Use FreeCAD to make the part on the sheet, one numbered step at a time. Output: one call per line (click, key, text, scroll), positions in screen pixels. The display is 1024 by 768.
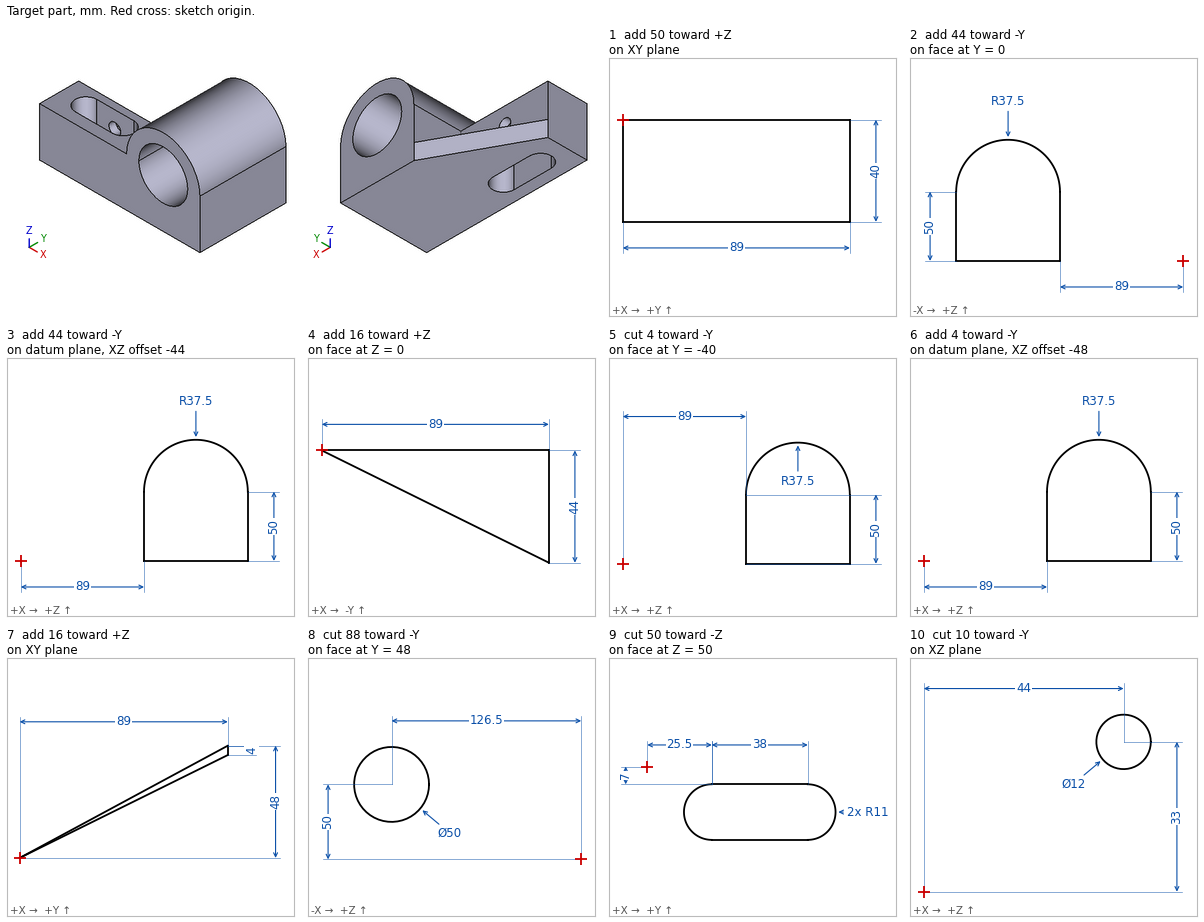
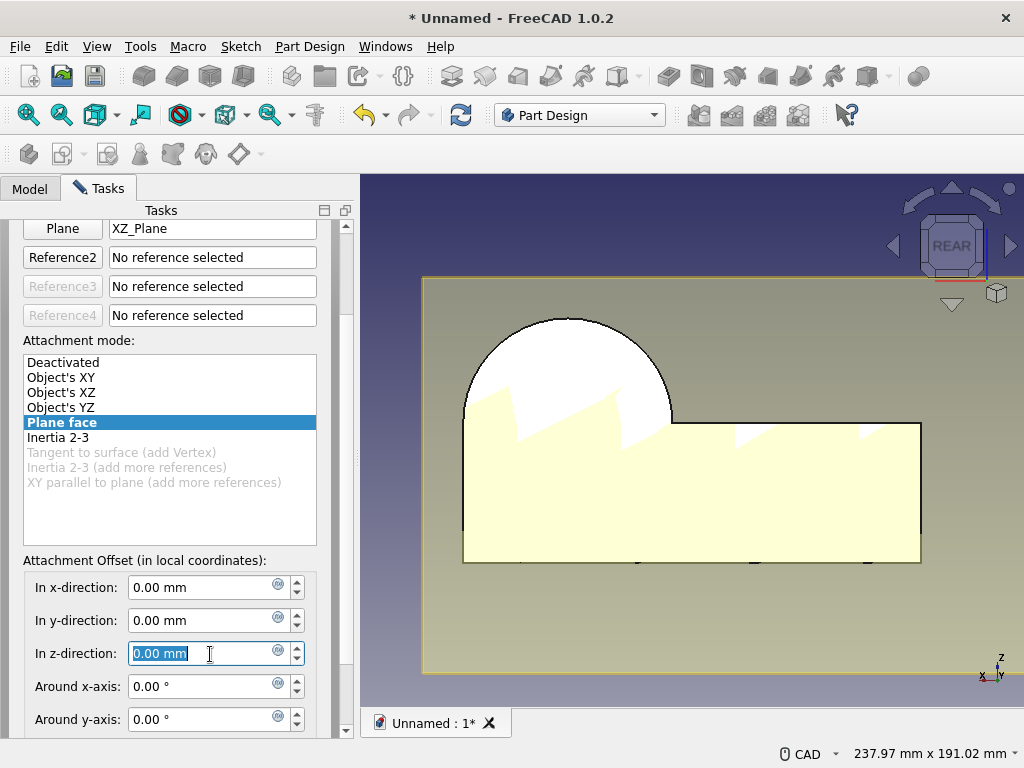
text(-44)
key(Tab)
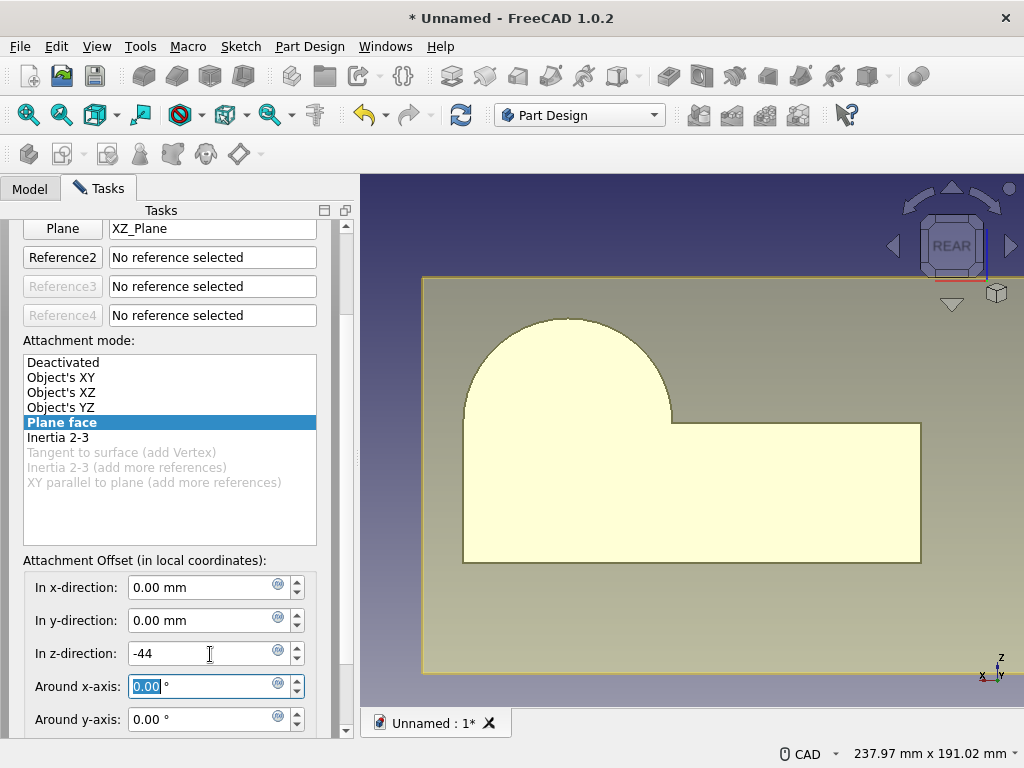
scroll(346, 479, up, 3)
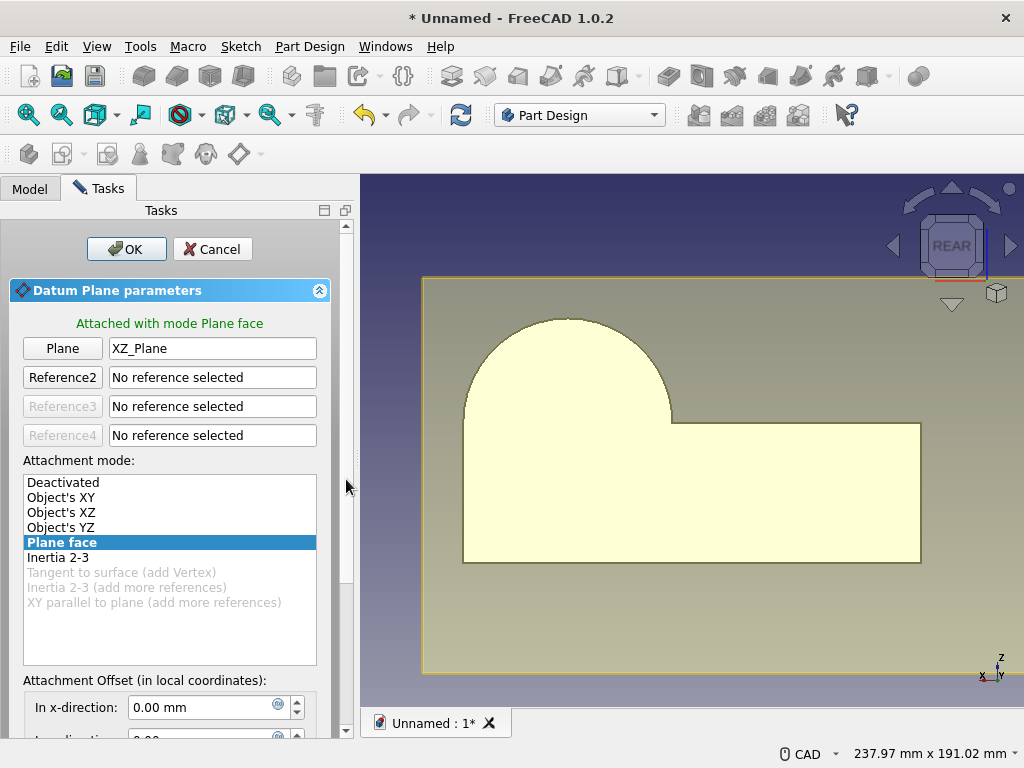
click(127, 249)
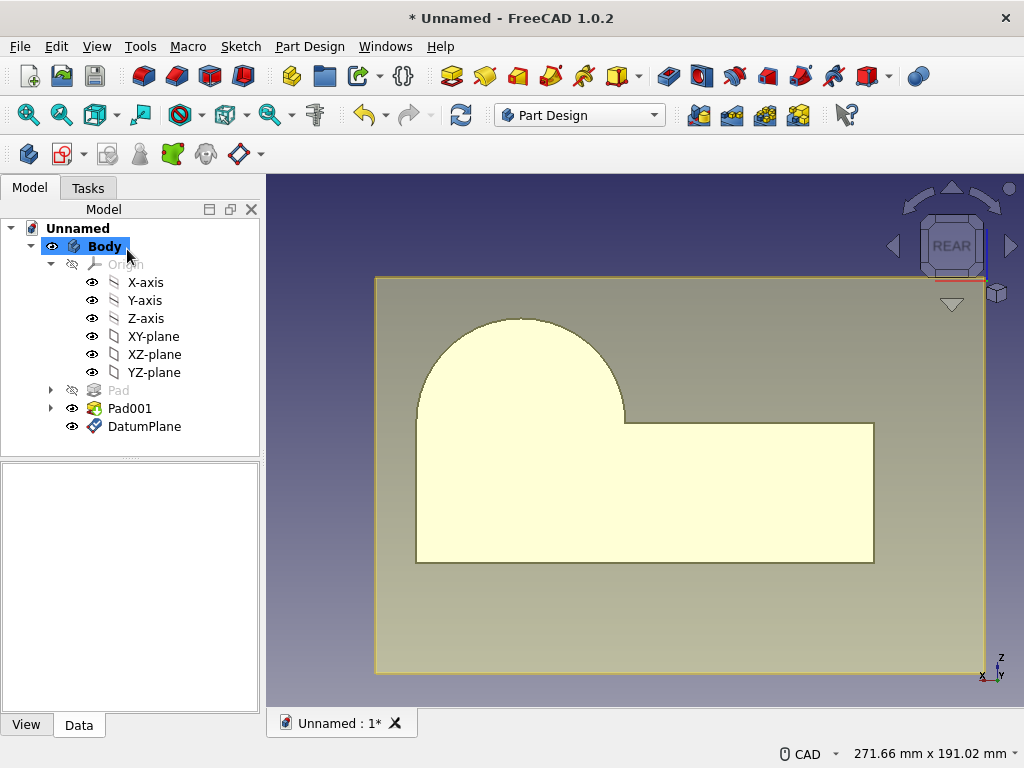
click(117, 426)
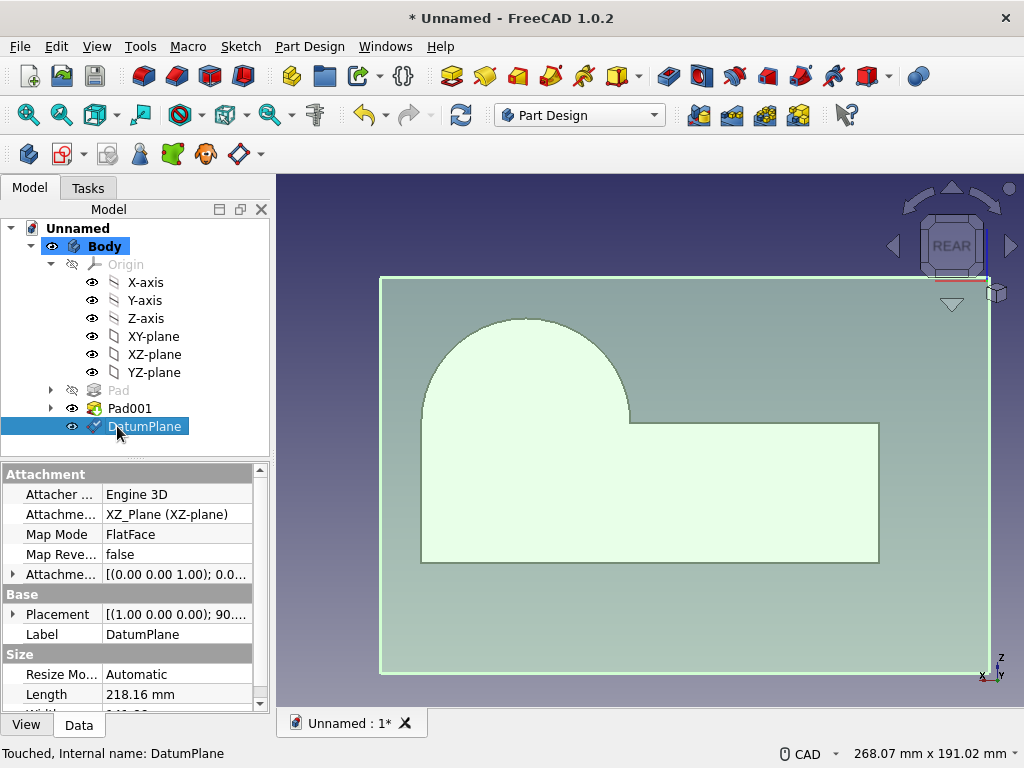
click(62, 154)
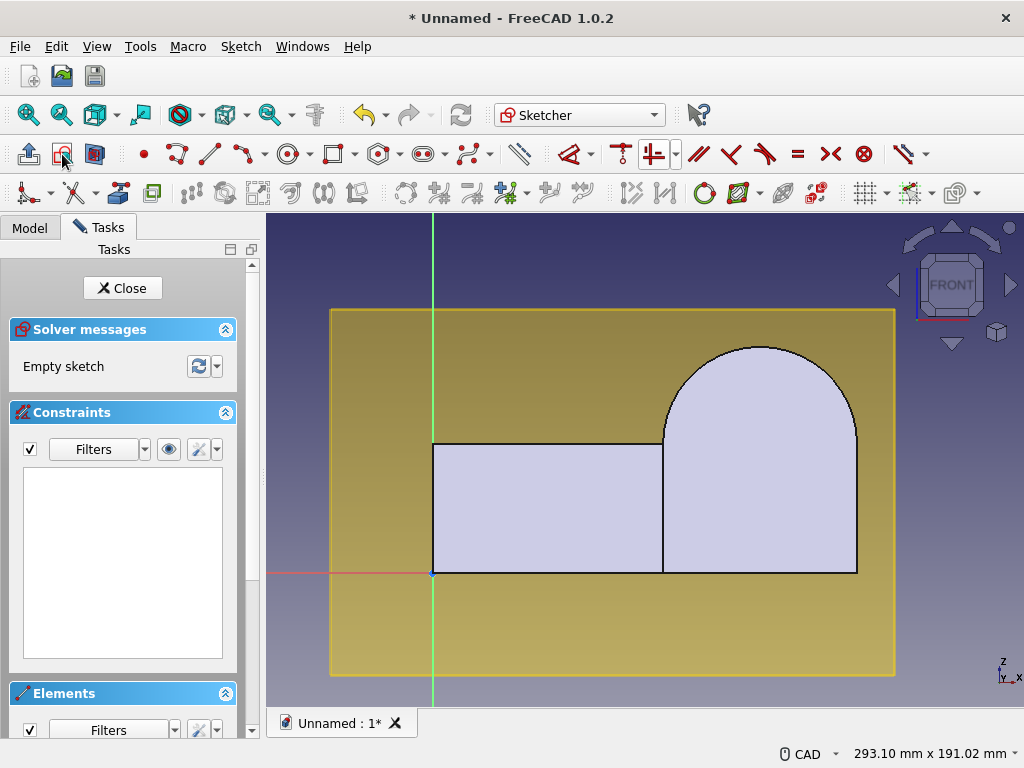
click(95, 154)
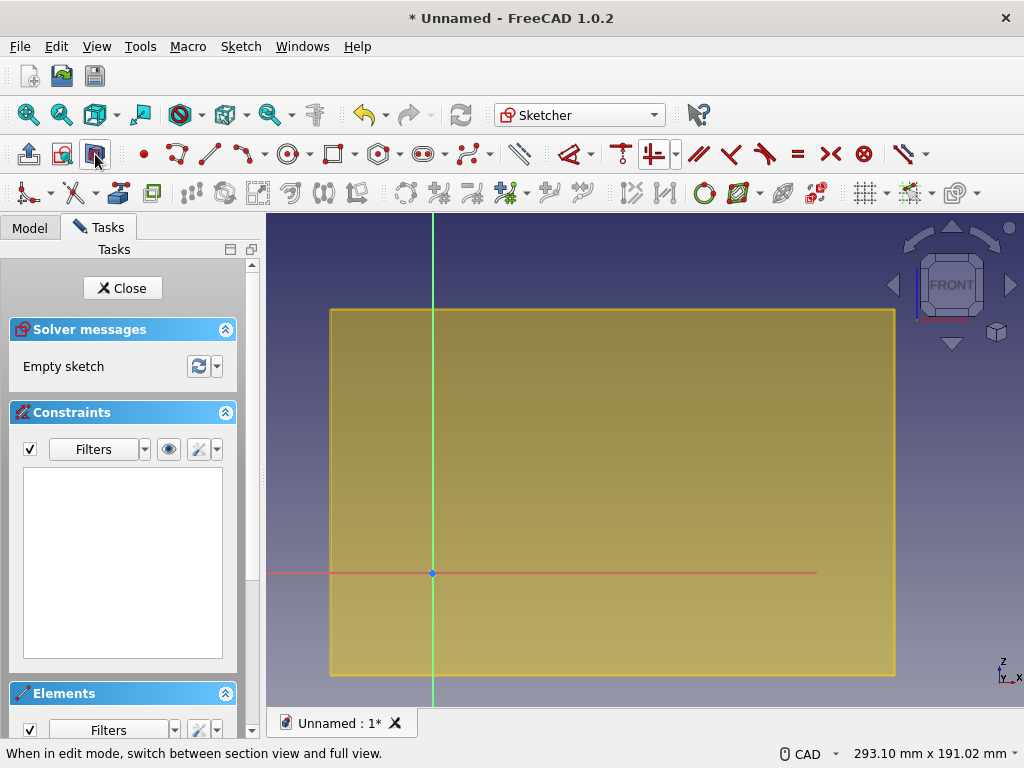
scroll(294, 460, down, 1)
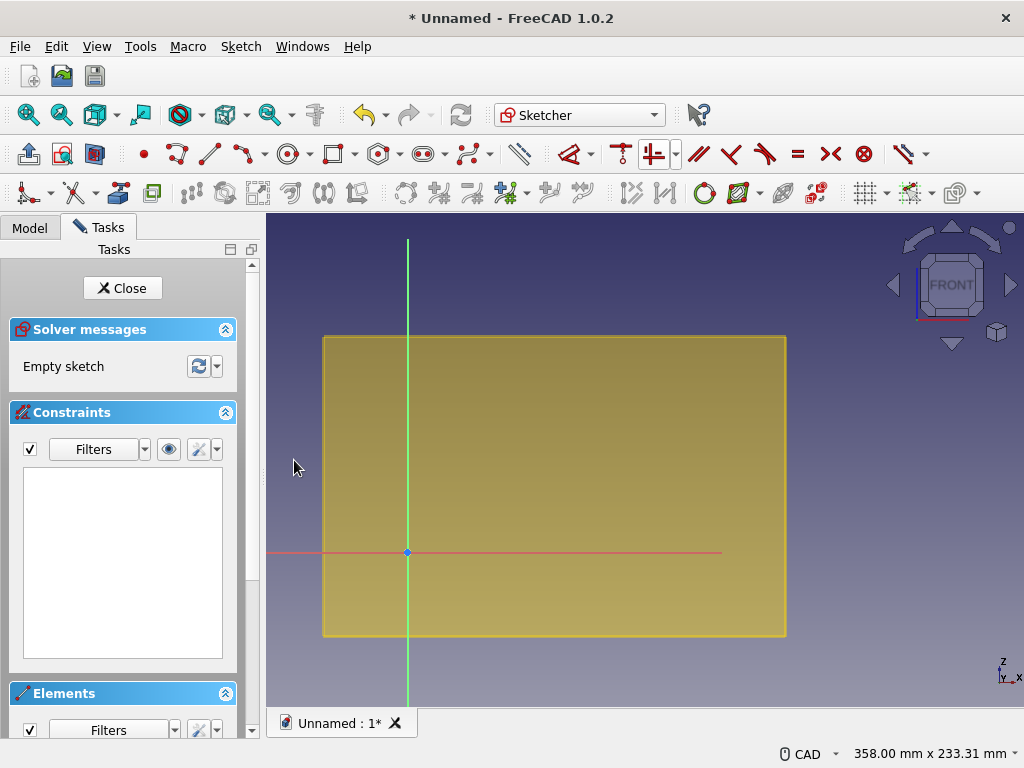
click(177, 154)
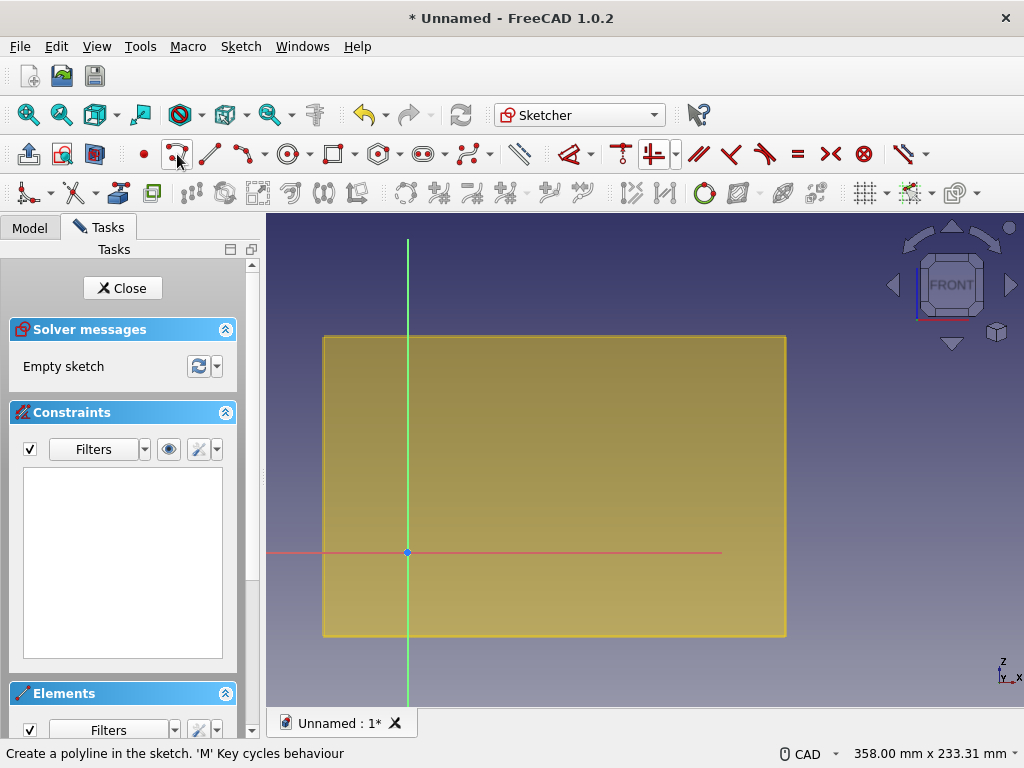
click(755, 447)
click(755, 553)
click(596, 544)
click(596, 447)
right_click(596, 447)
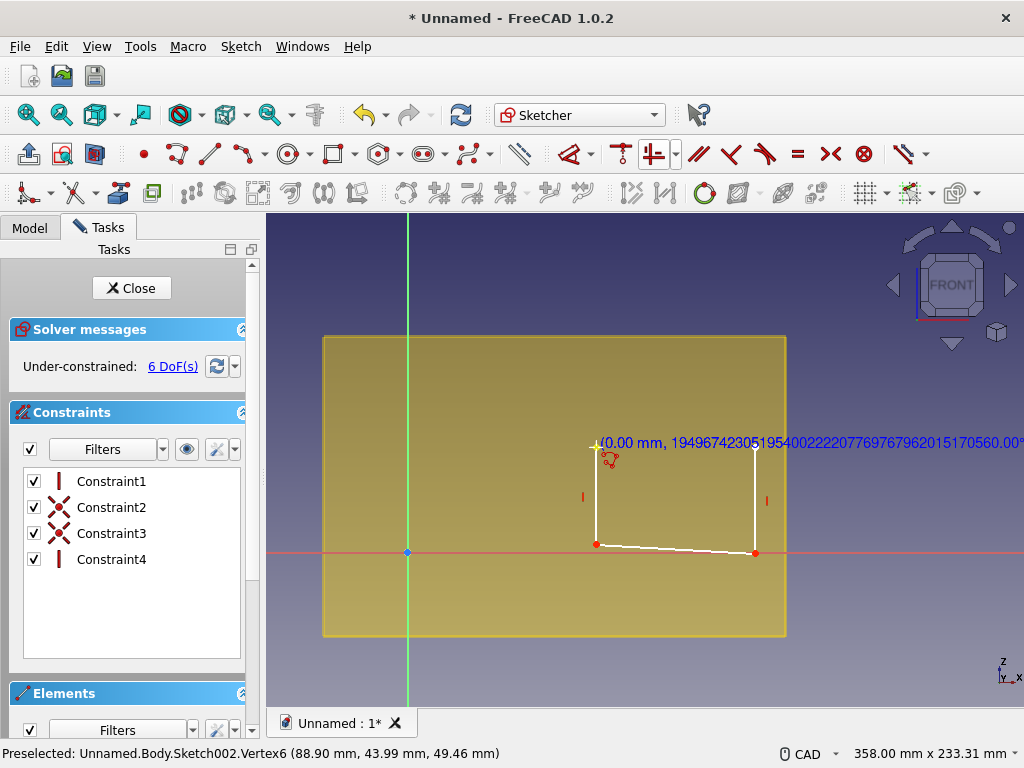
key(g)
key(3)
key(a)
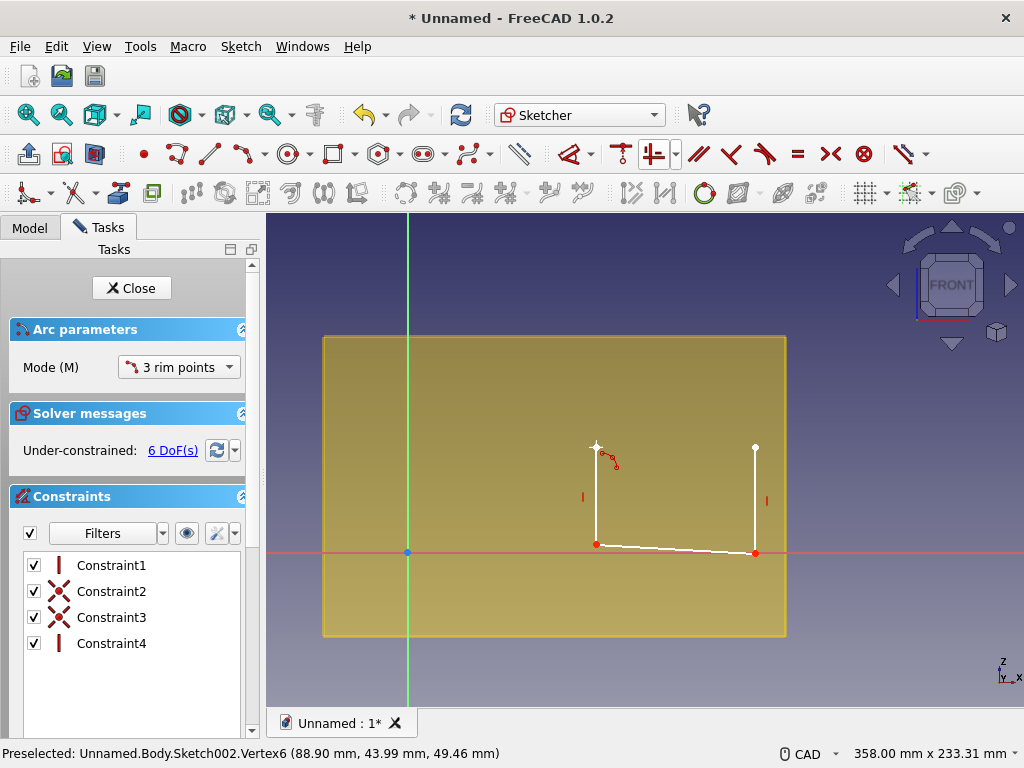
click(596, 448)
click(755, 448)
click(676, 367)
key(Escape)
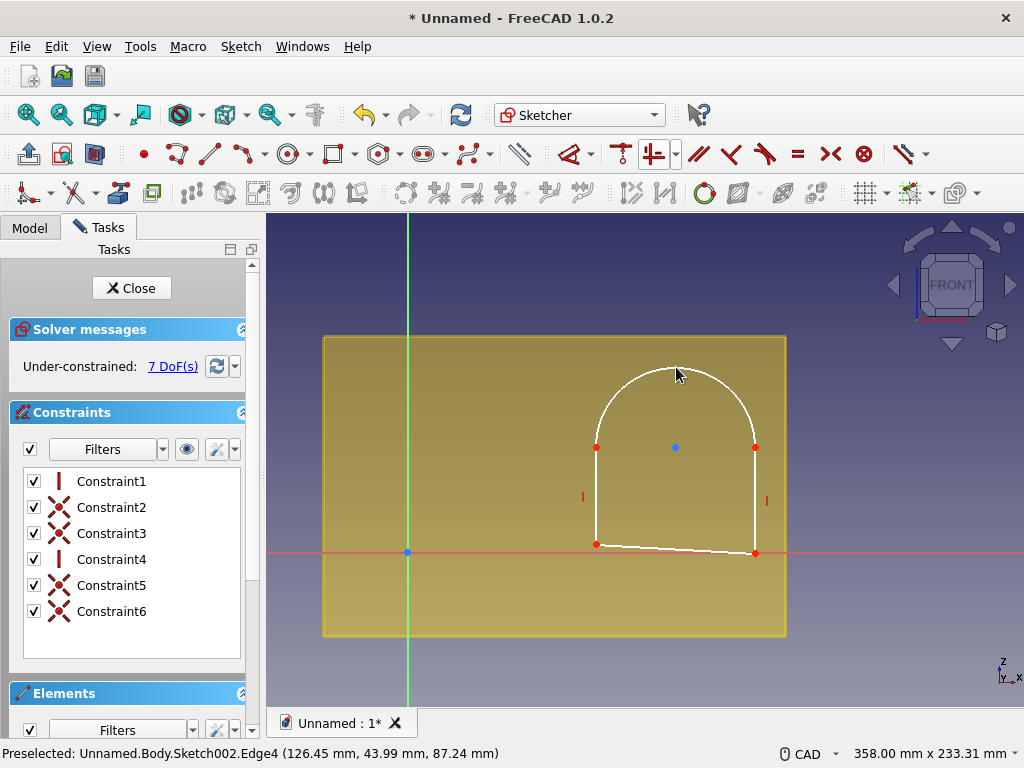
click(755, 480)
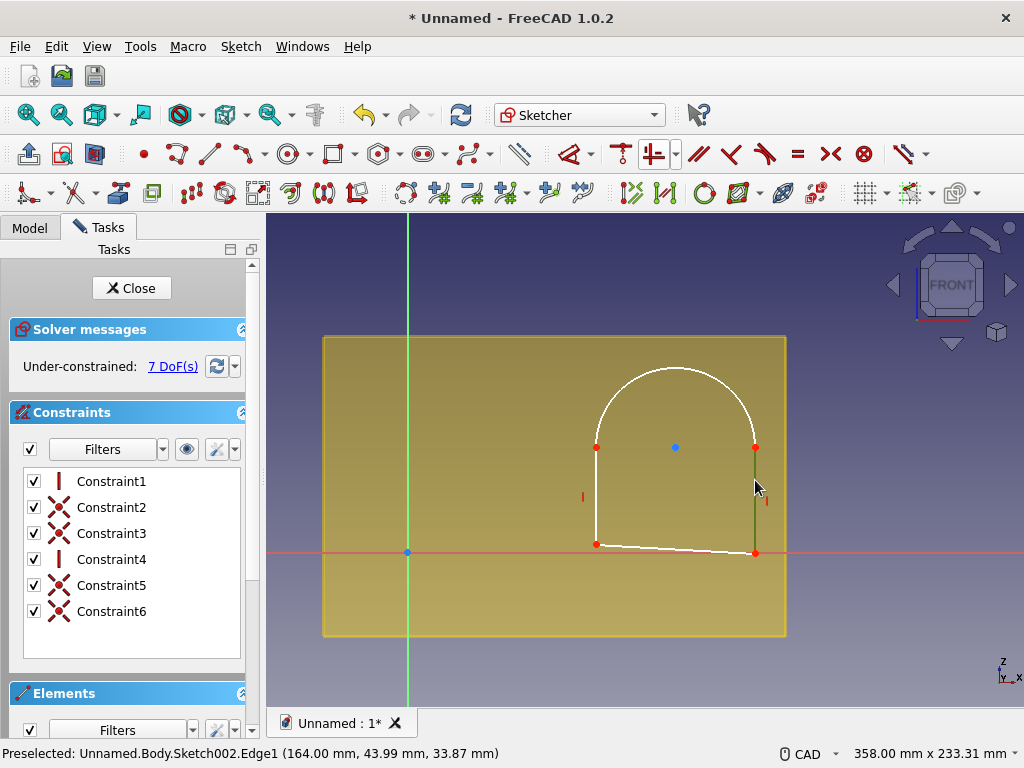
click(722, 383)